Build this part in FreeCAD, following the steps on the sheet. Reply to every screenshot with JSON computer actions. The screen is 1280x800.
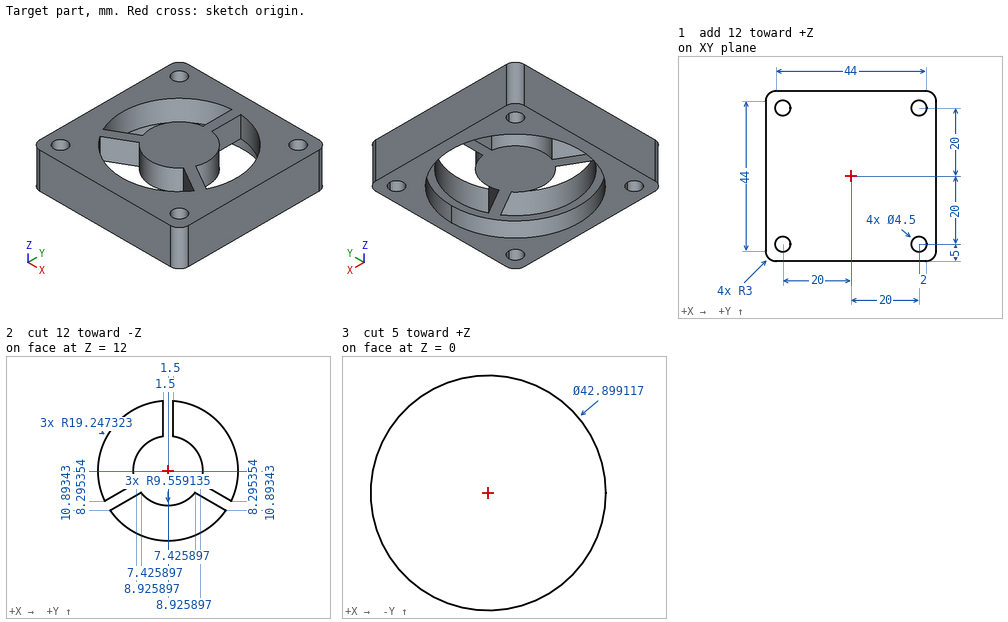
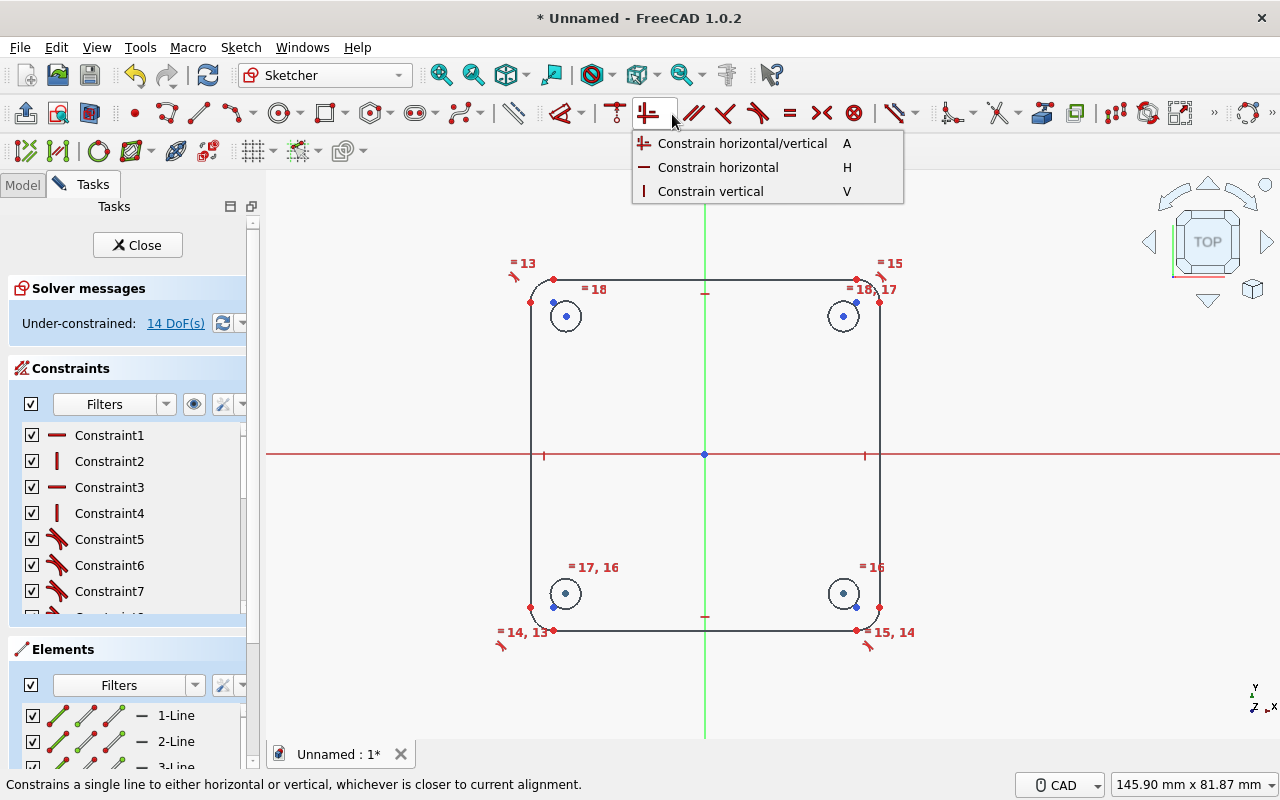
{"action": "left_click", "coordinate": [768, 167]}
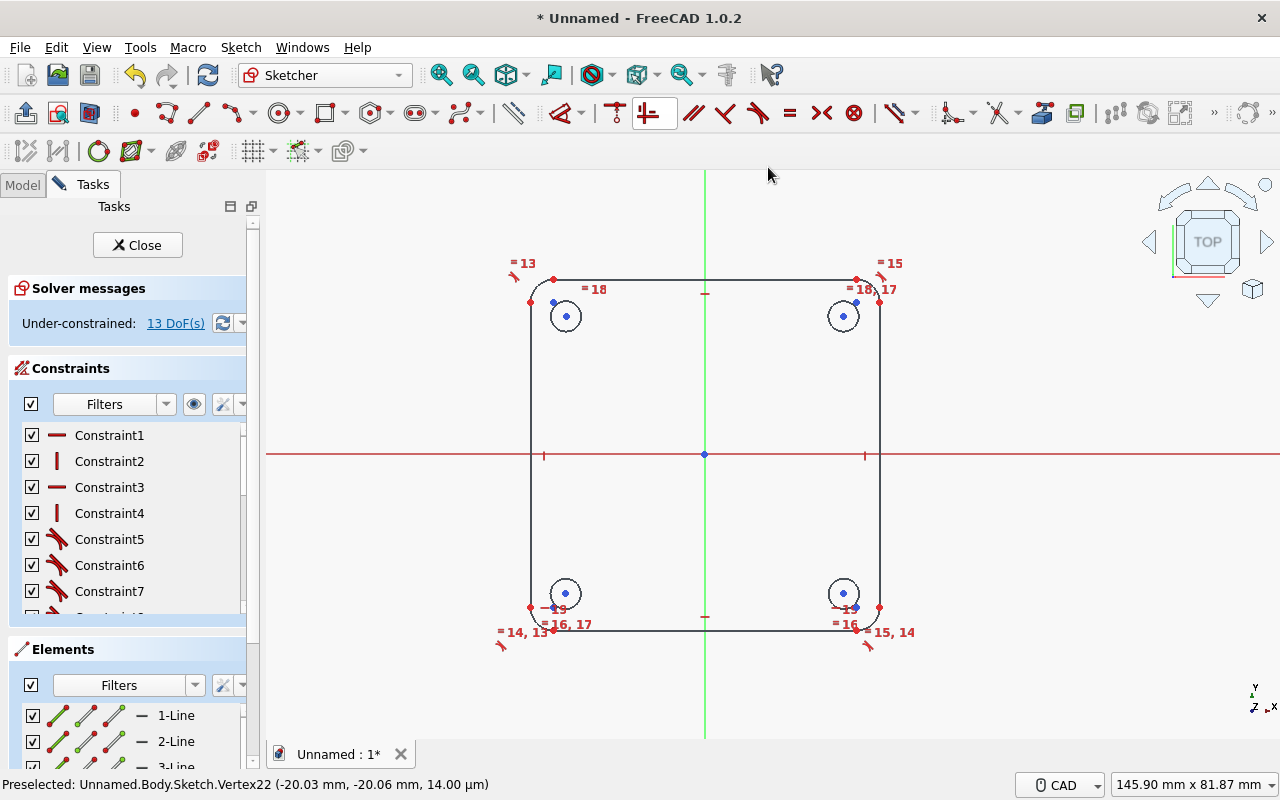
{"action": "left_click", "coordinate": [844, 594]}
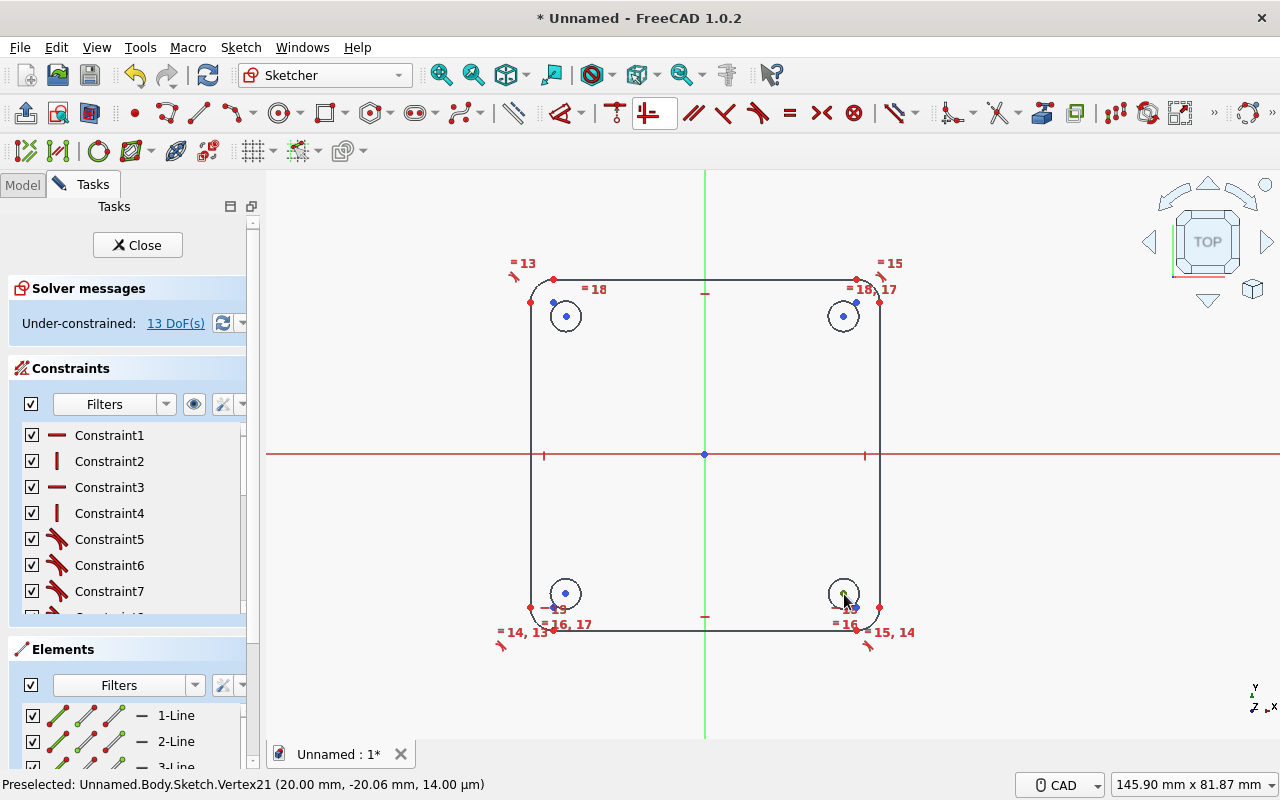
{"action": "left_click", "coordinate": [844, 316]}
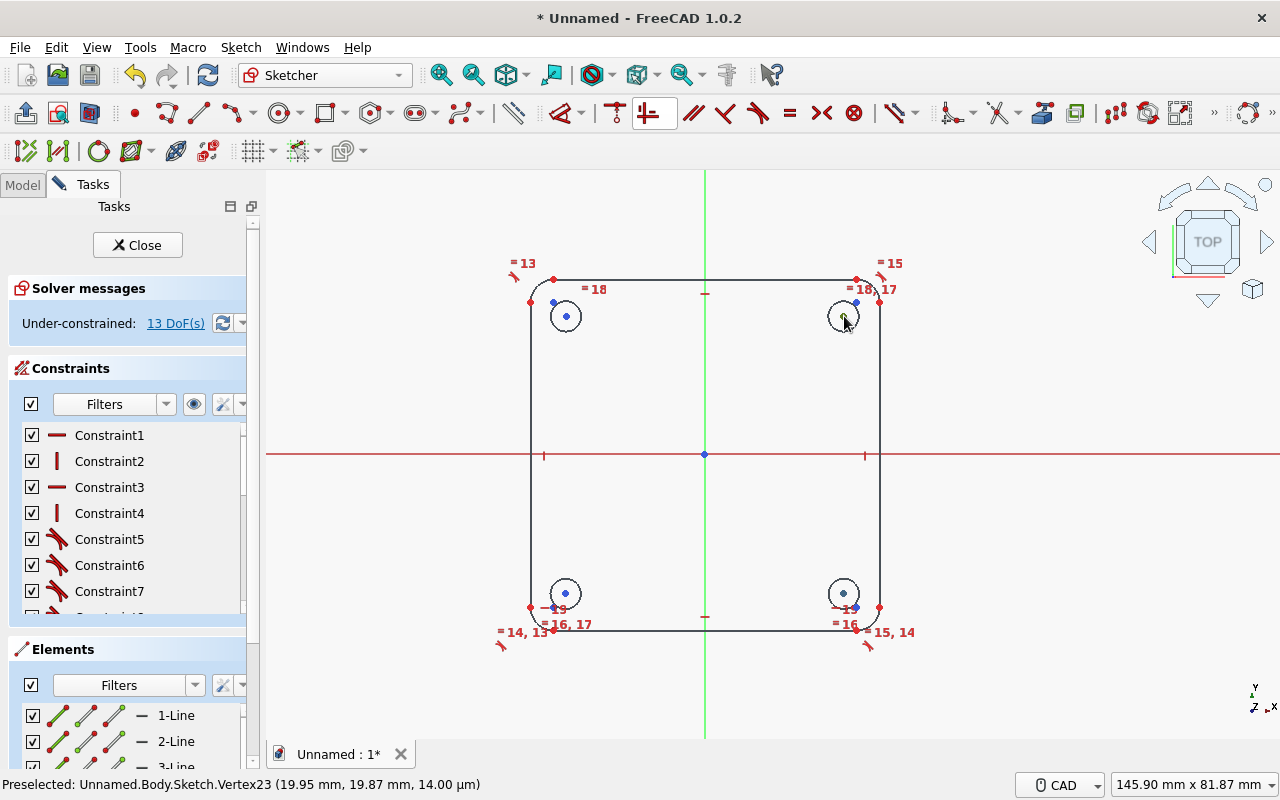
{"action": "left_click", "coordinate": [672, 114]}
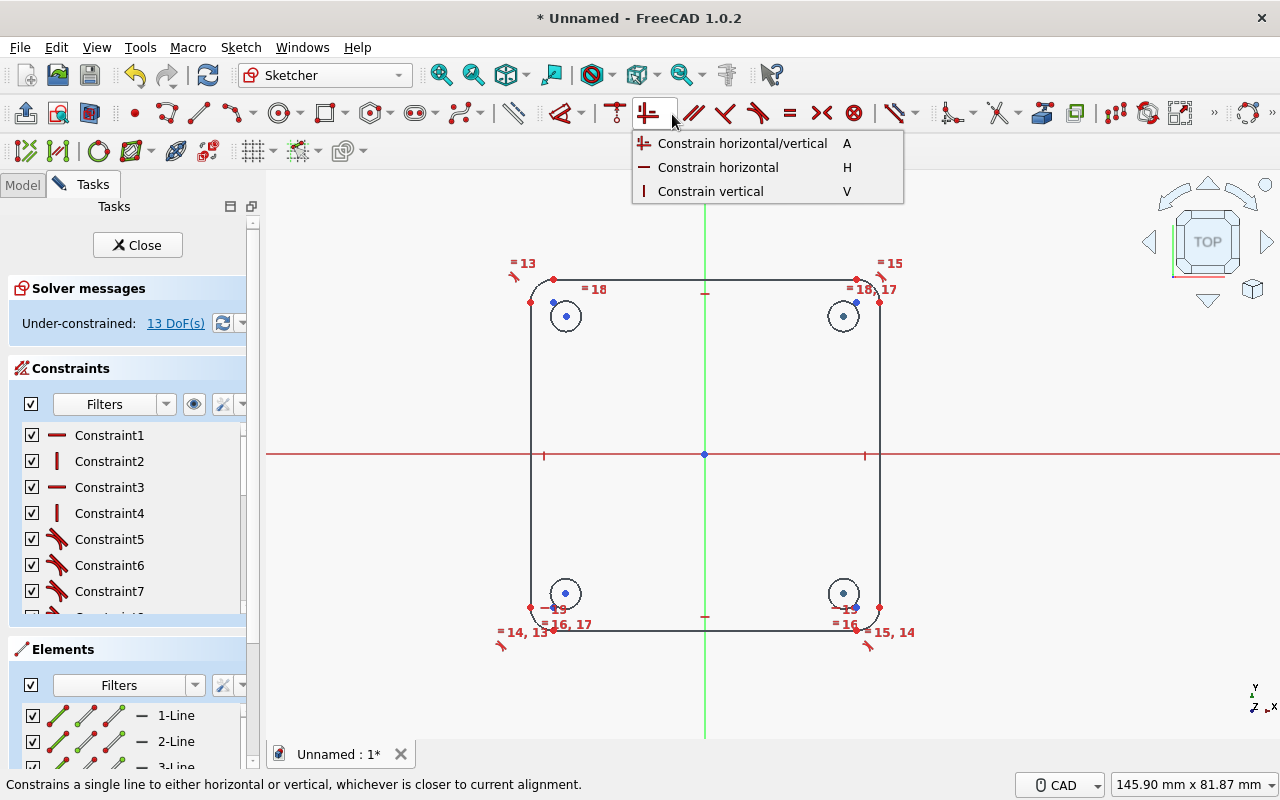
{"action": "left_click", "coordinate": [768, 191]}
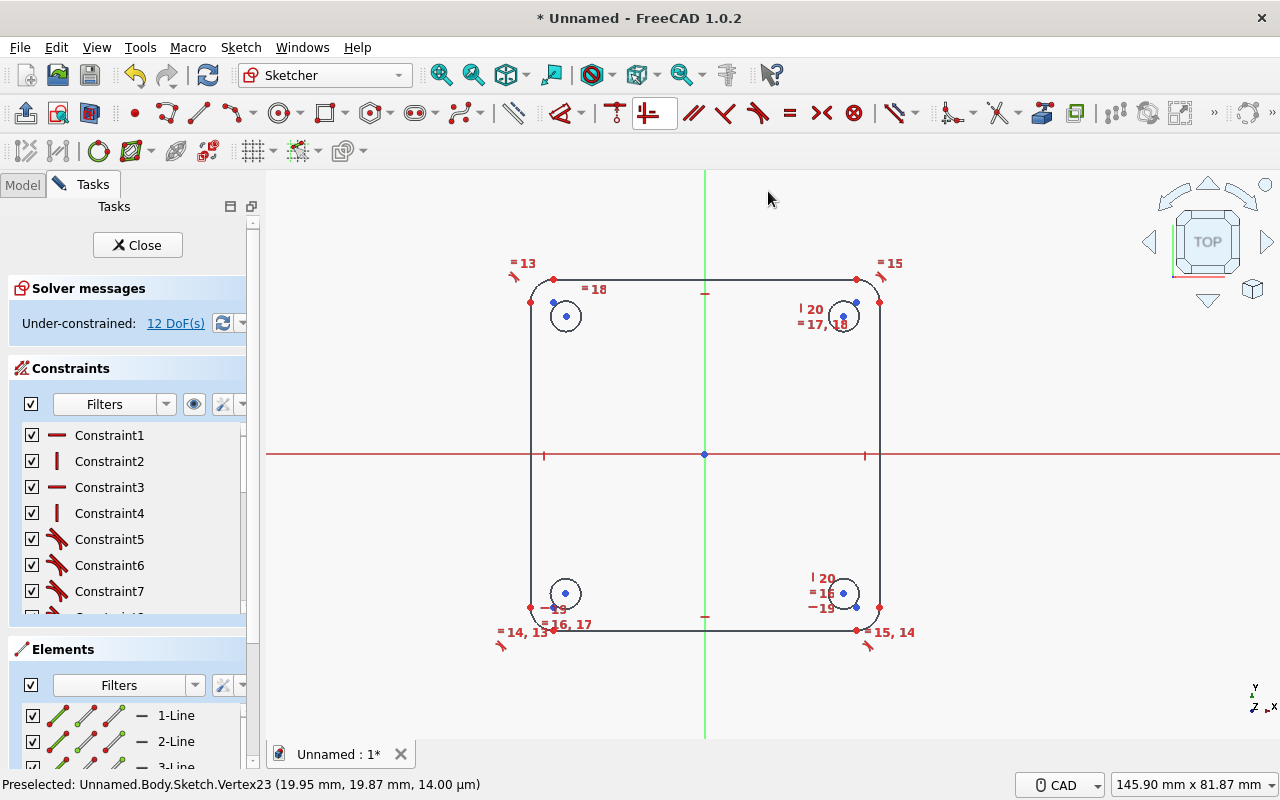
{"action": "left_click", "coordinate": [566, 594]}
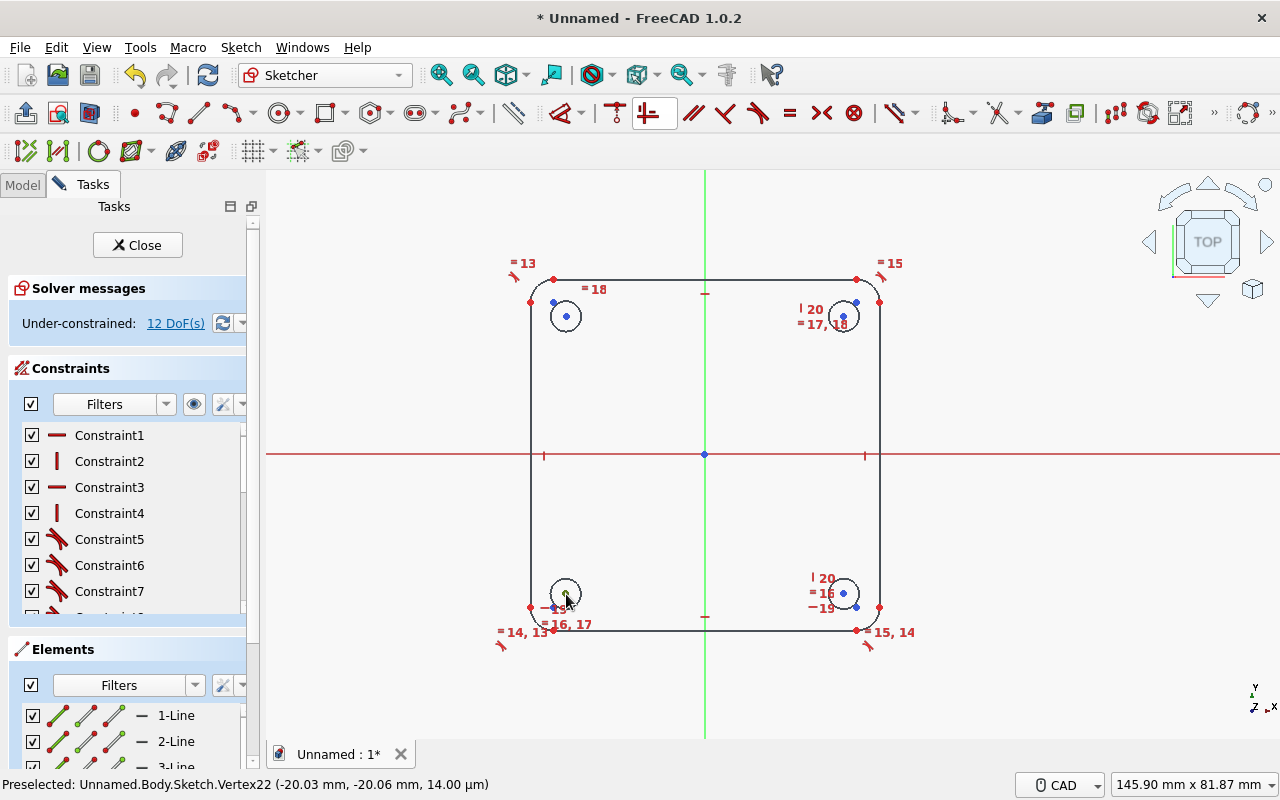
{"action": "left_click", "coordinate": [566, 316]}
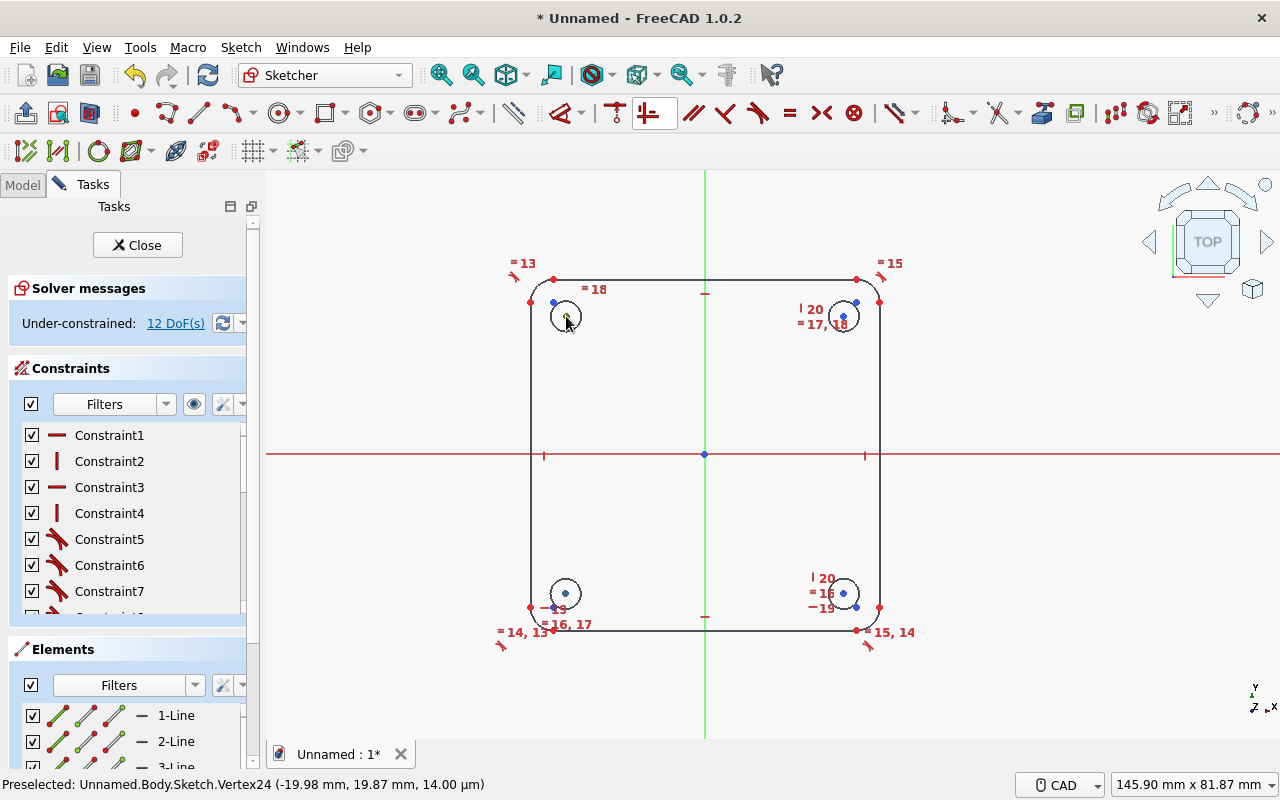
{"action": "key", "text": "v"}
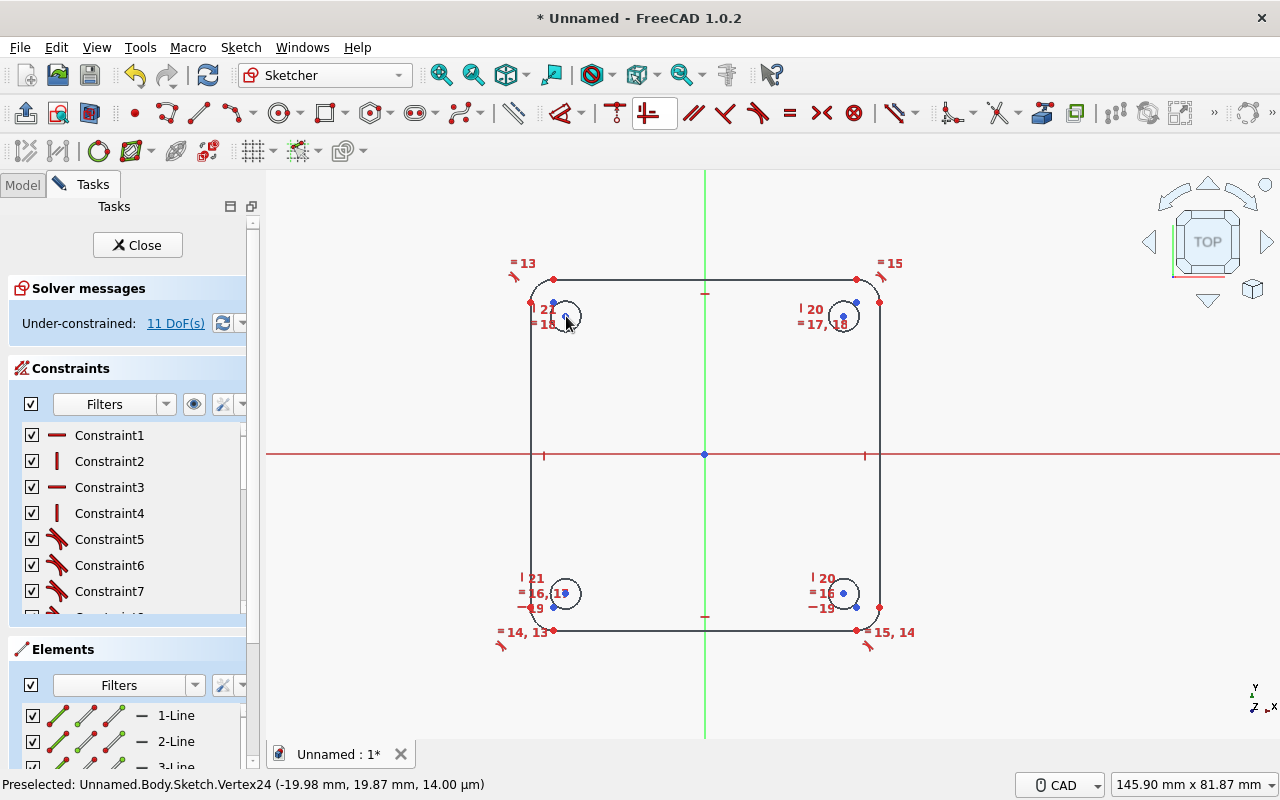
{"action": "scroll", "coordinate": [844, 316], "scroll_direction": "up", "scroll_amount": 4}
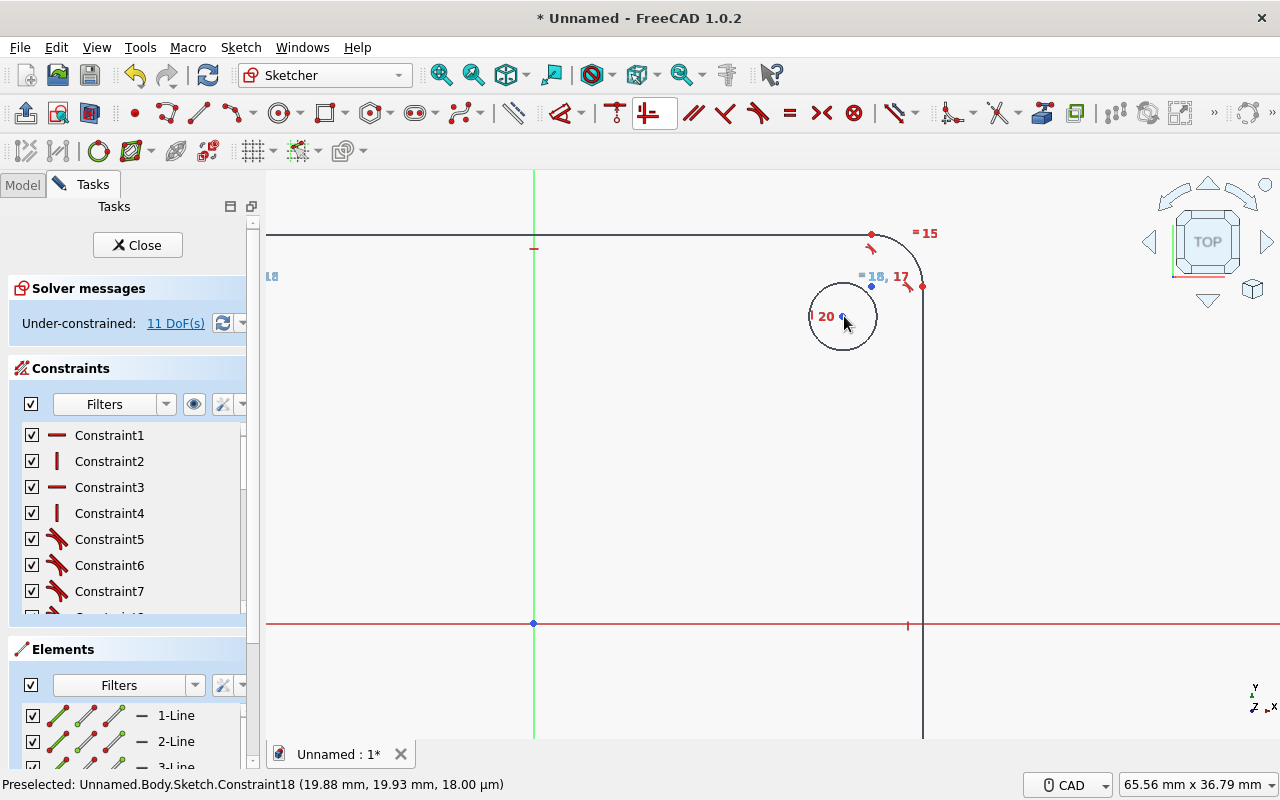
{"action": "left_click", "coordinate": [843, 317]}